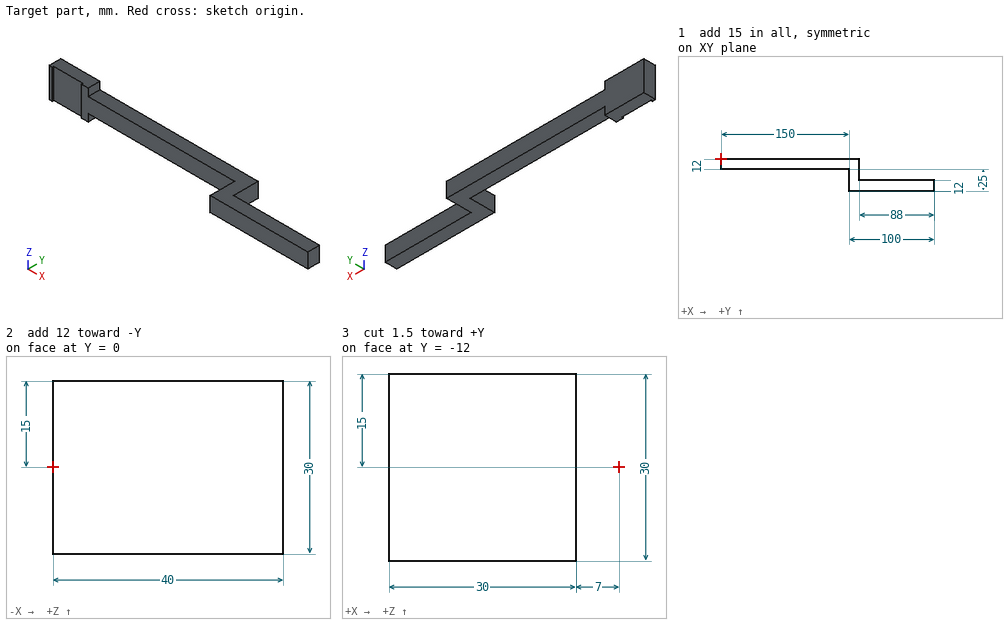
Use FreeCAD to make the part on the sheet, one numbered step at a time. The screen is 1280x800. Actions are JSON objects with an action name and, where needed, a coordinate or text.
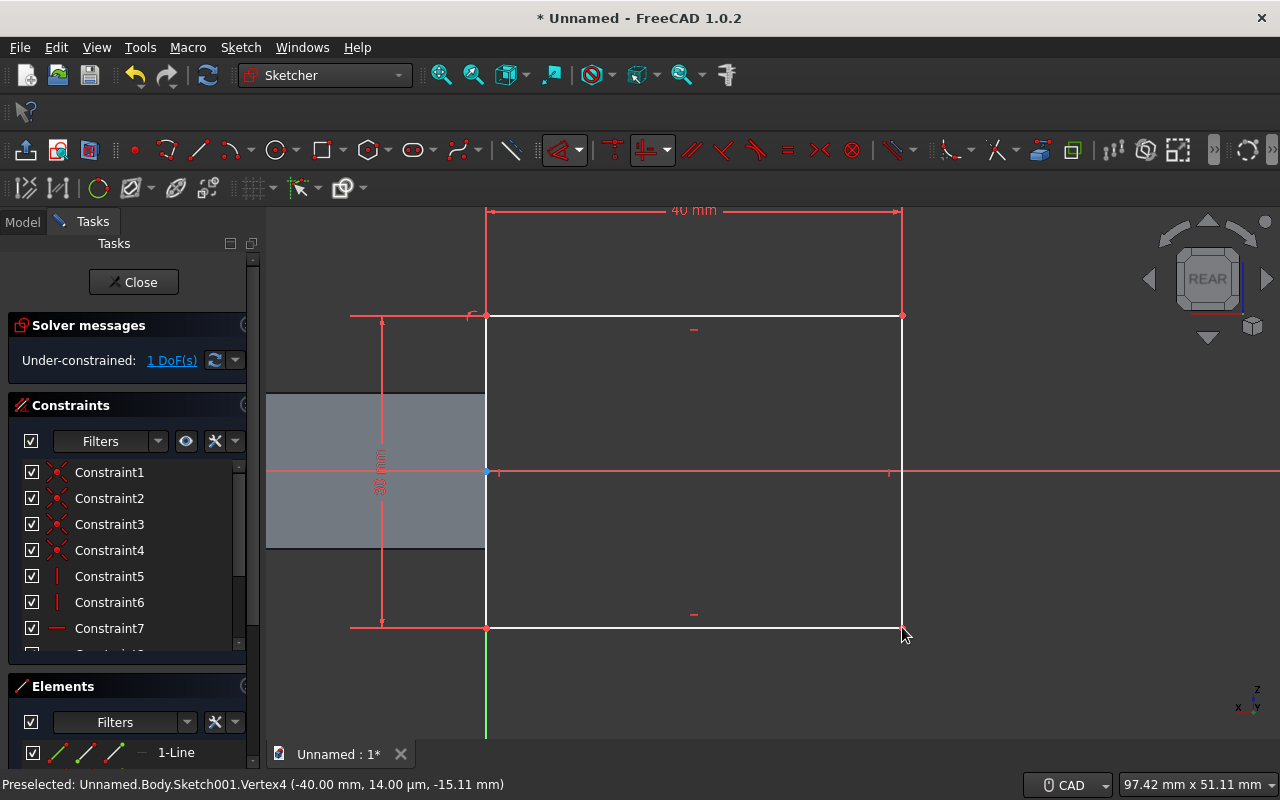
{"action": "left_click", "coordinate": [486, 316]}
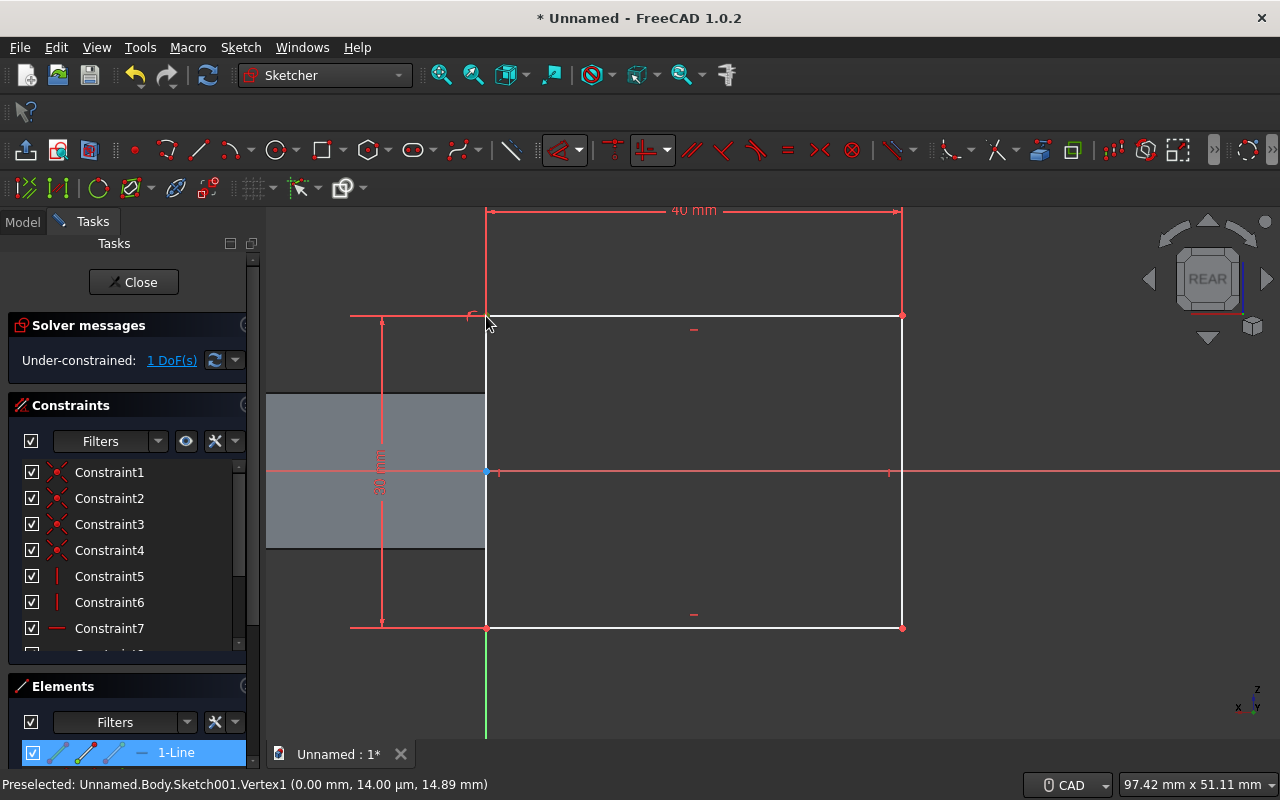
{"action": "left_click", "coordinate": [582, 150]}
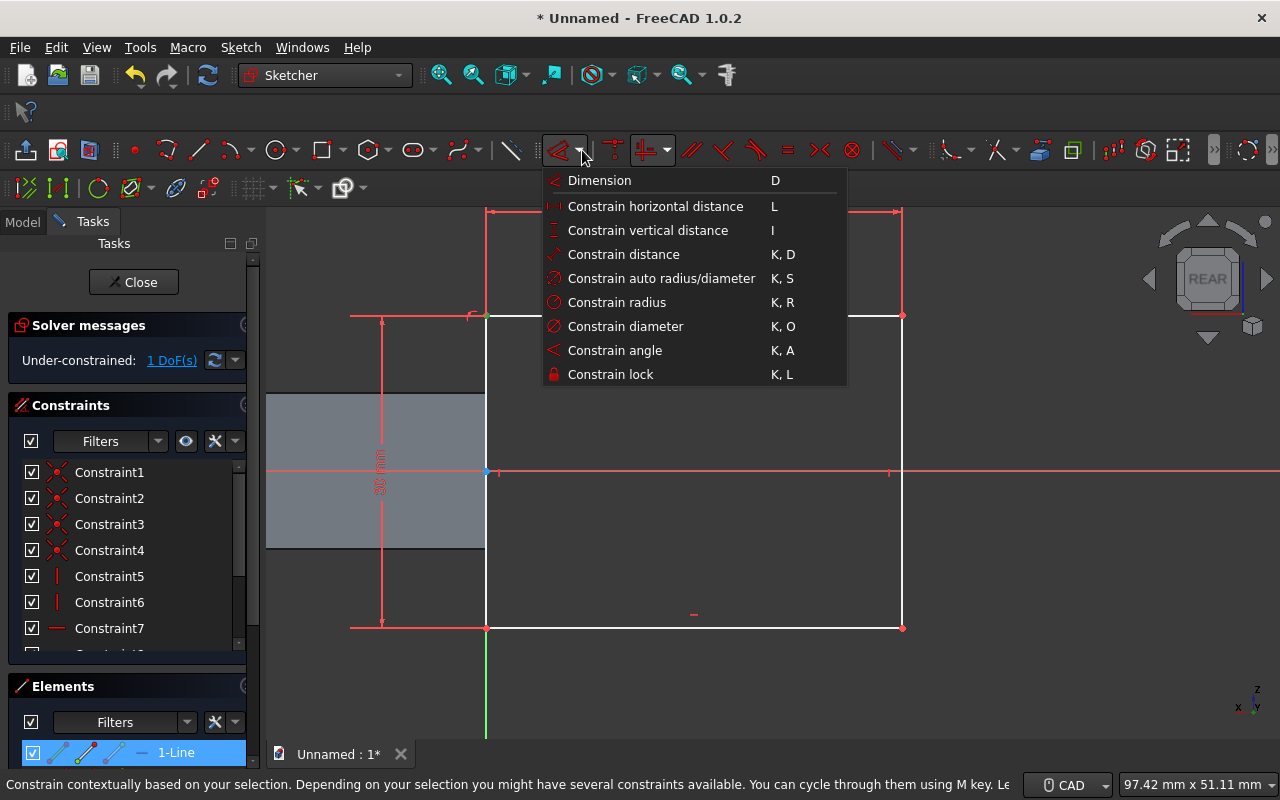
{"action": "left_click", "coordinate": [695, 230]}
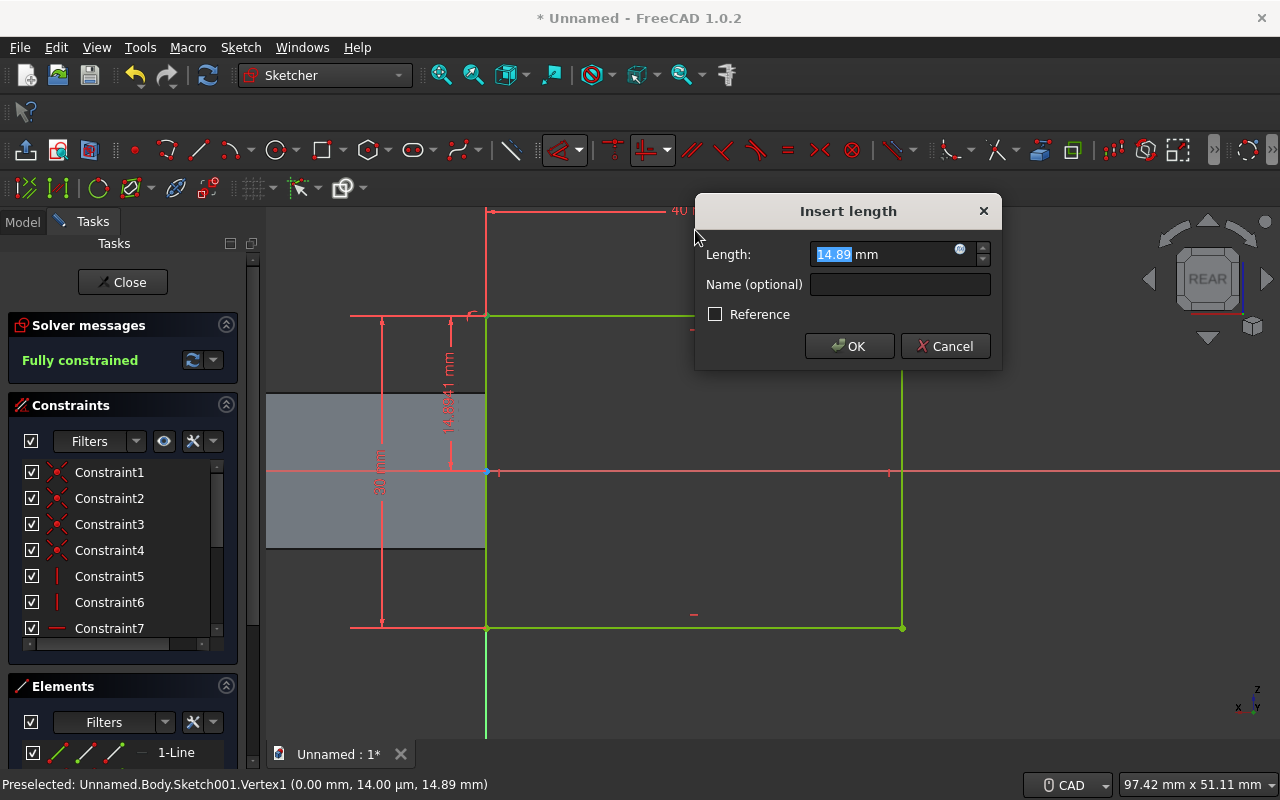
{"action": "type", "text": "15"}
{"action": "key", "text": "Return"}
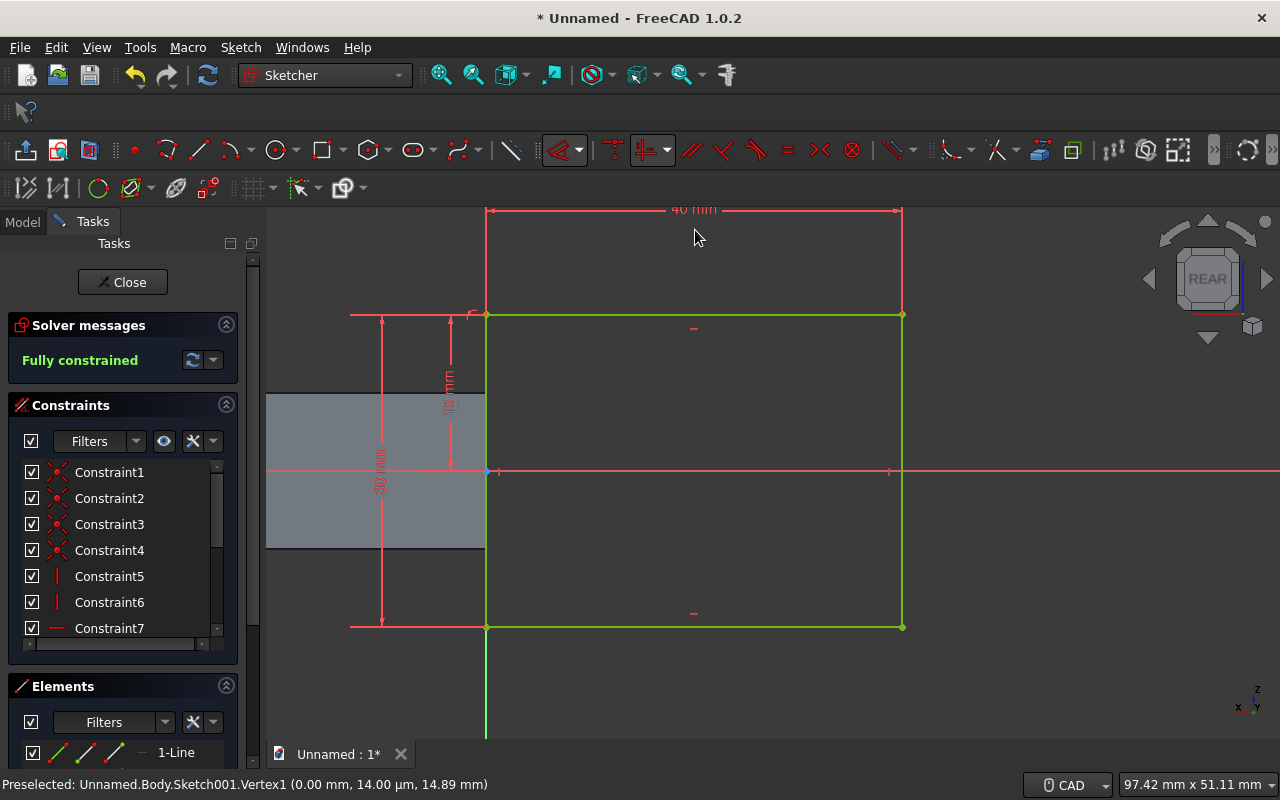
{"action": "left_click", "coordinate": [123, 282]}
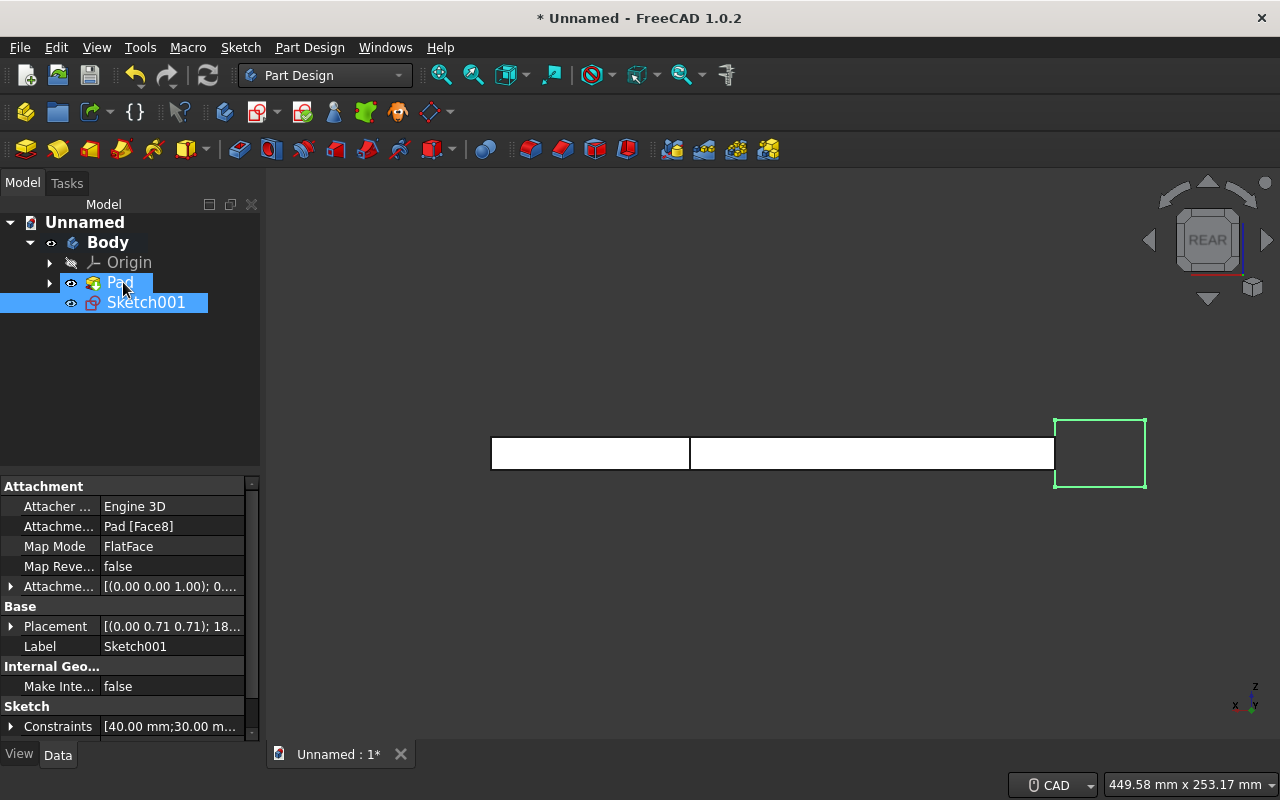
{"action": "left_click", "coordinate": [26, 150]}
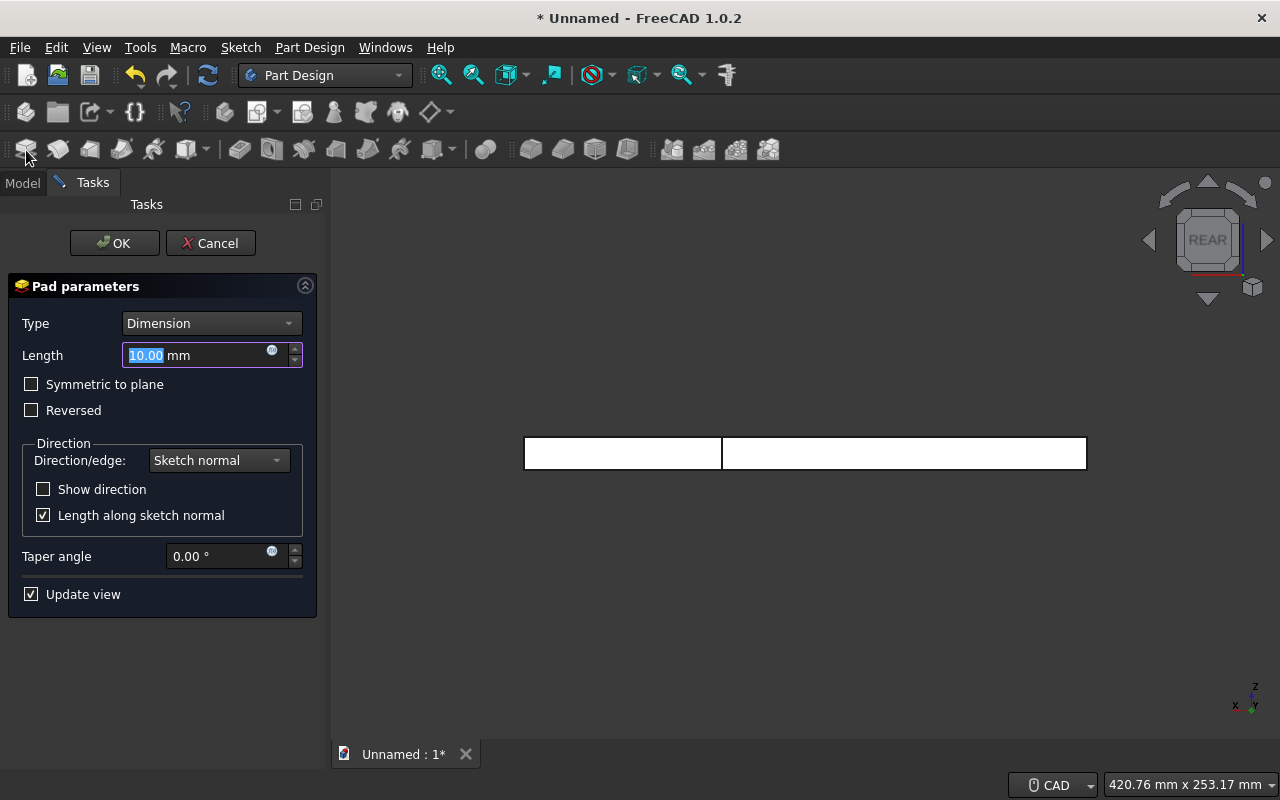
{"action": "type", "text": "12"}
{"action": "key", "text": "Tab"}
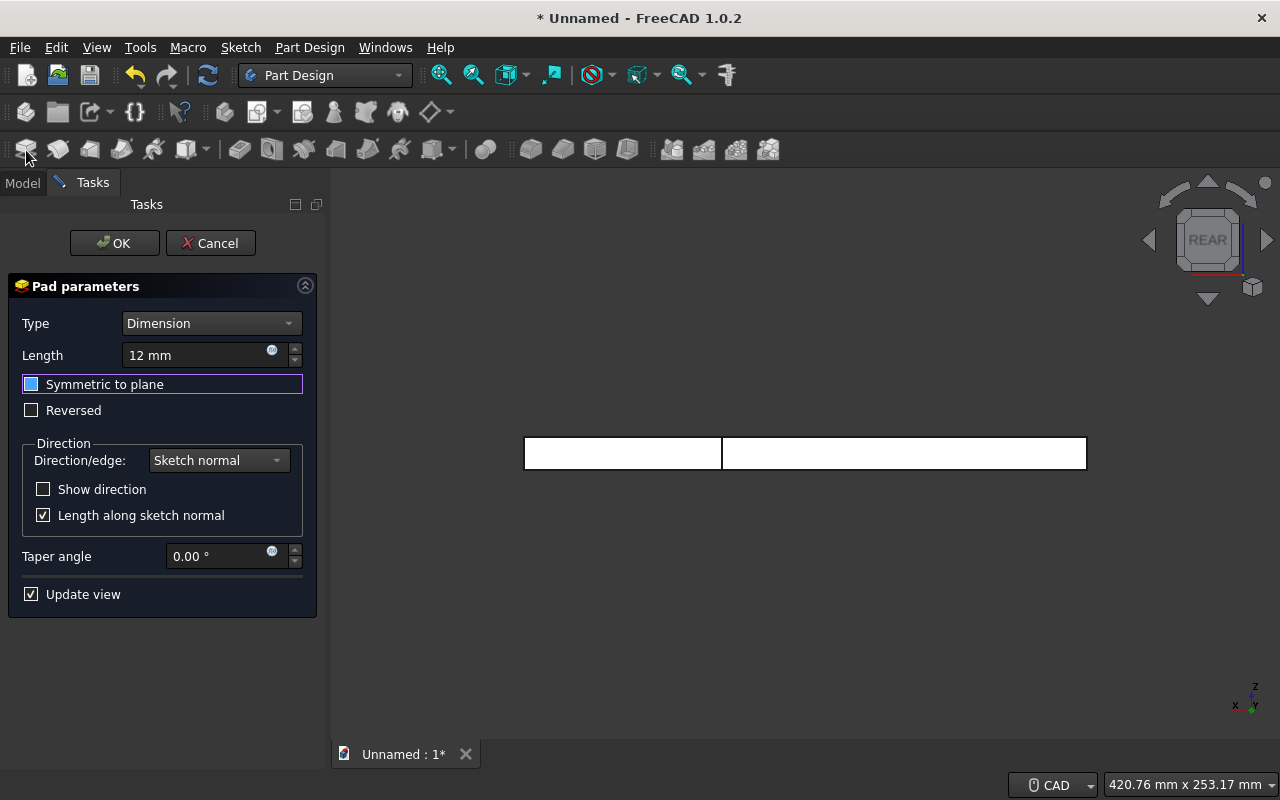
{"action": "left_click", "coordinate": [30, 410]}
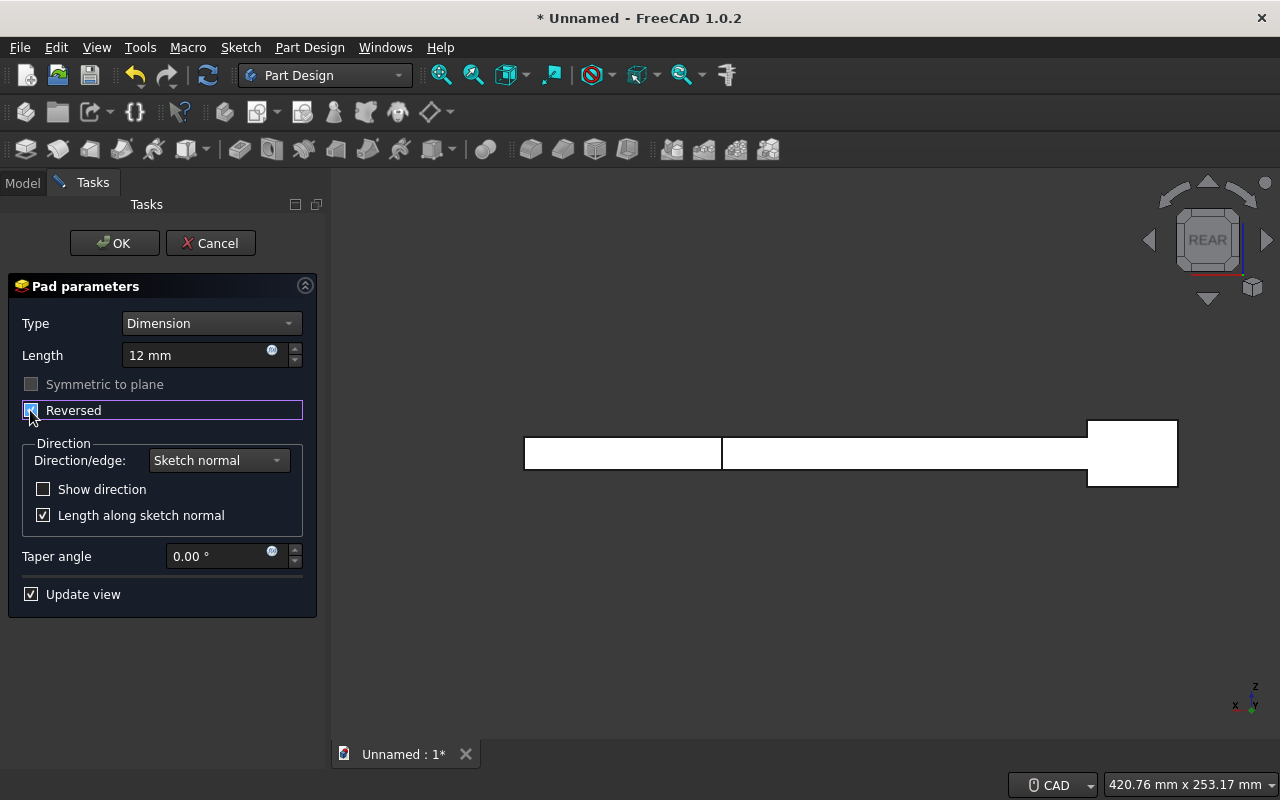
{"action": "left_click", "coordinate": [115, 243]}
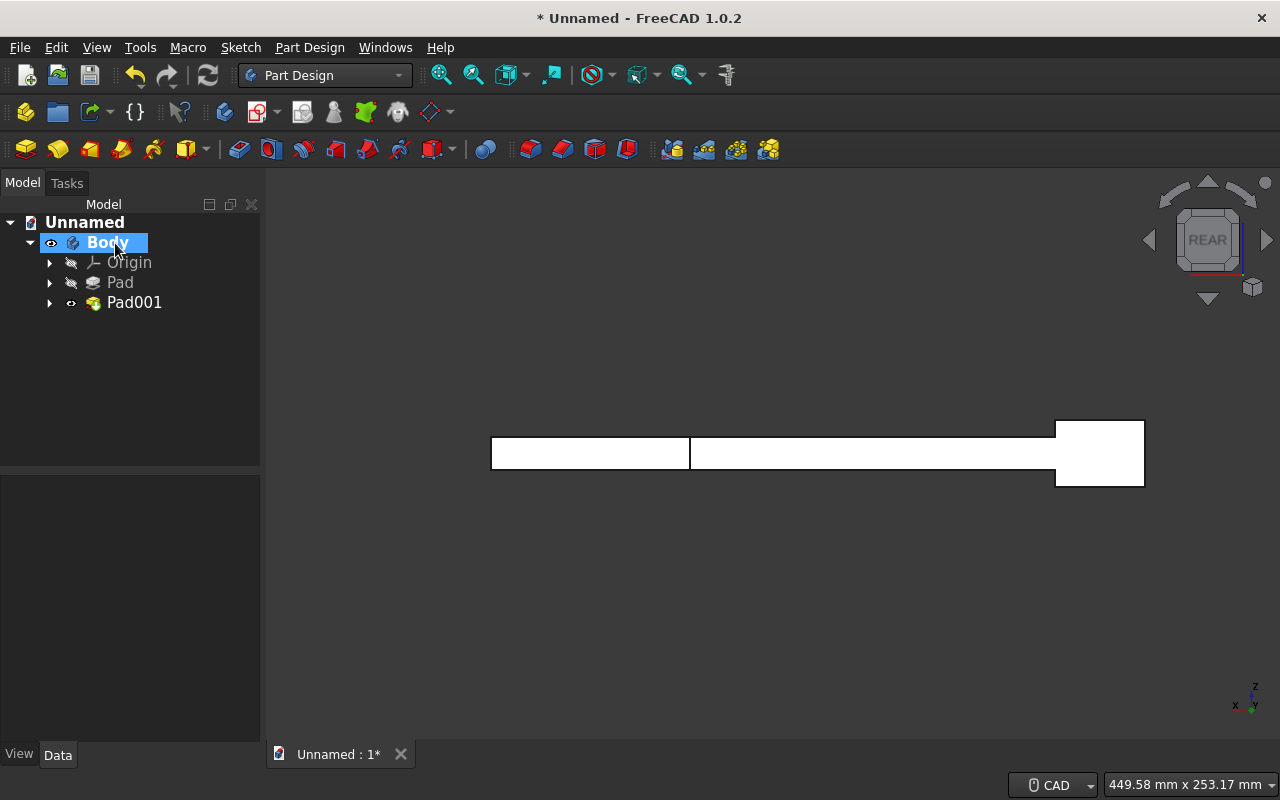
{"action": "key", "text": "0"}